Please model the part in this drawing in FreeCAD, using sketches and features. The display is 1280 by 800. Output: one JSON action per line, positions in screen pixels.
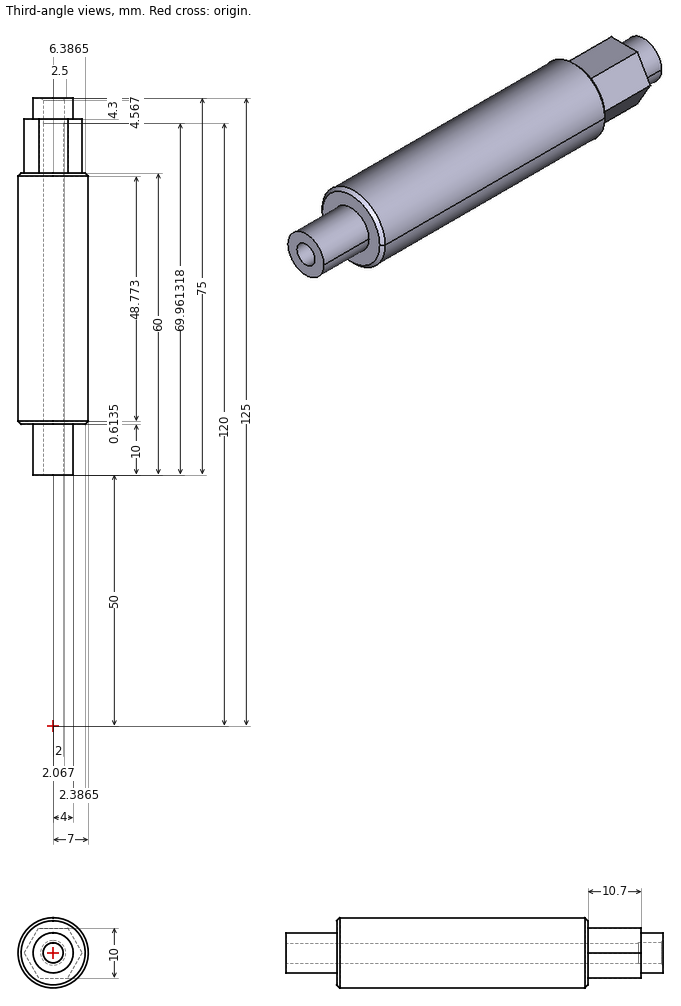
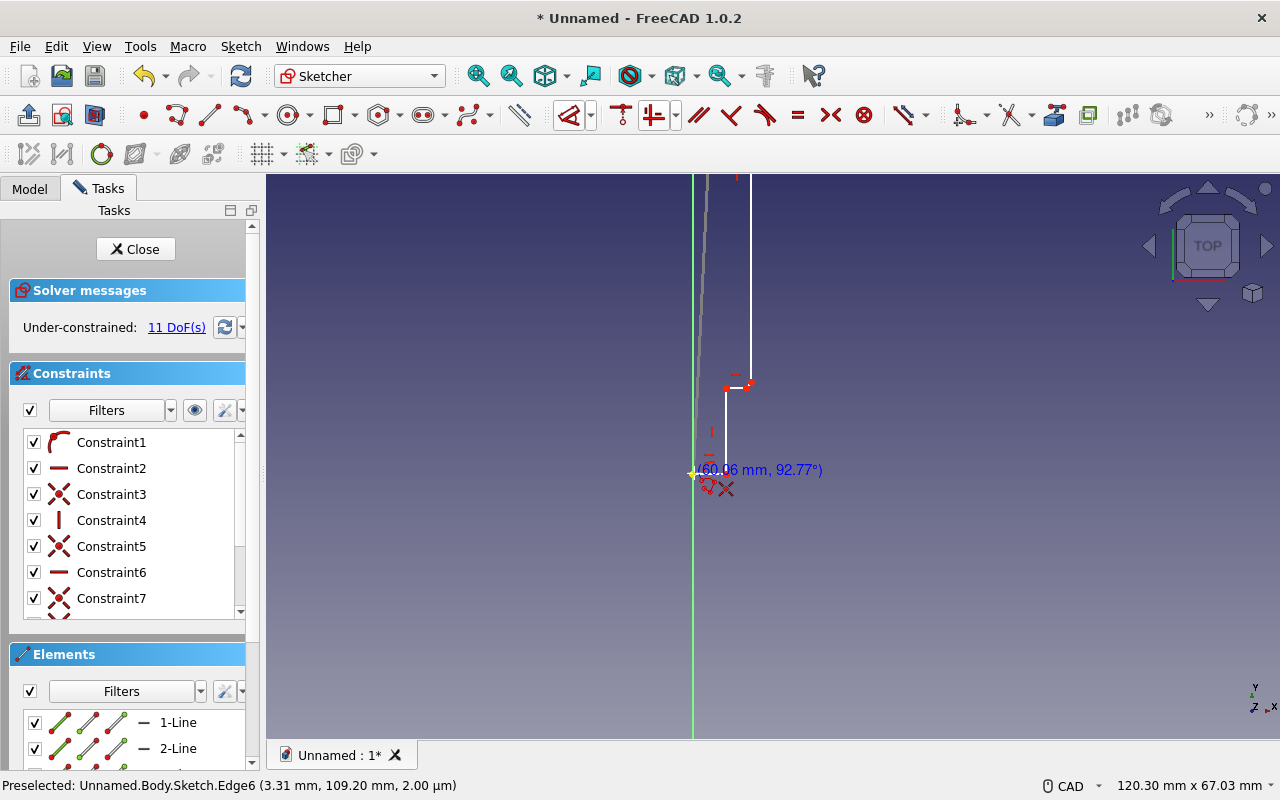
{"action": "left_click", "coordinate": [693, 474]}
{"action": "key", "text": "Escape"}
{"action": "key", "text": "Escape"}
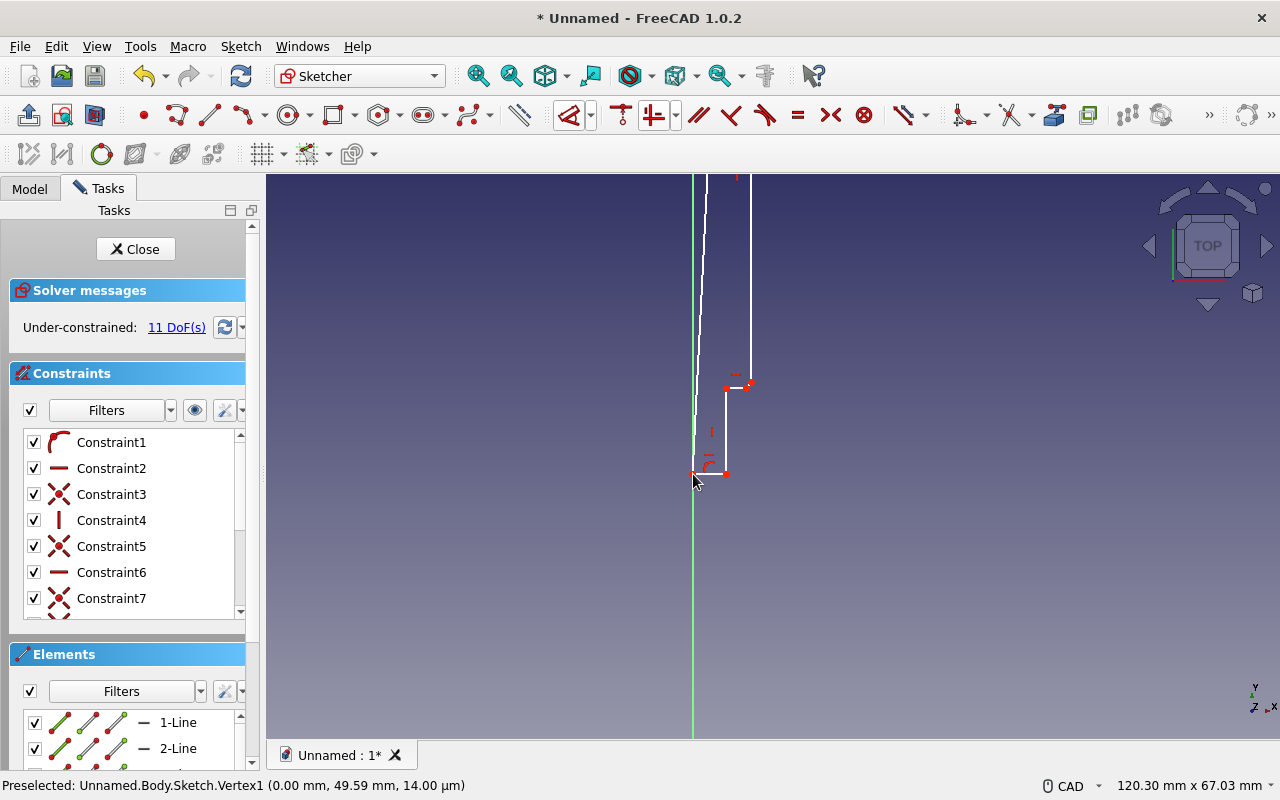
{"action": "scroll", "coordinate": [694, 473], "scroll_direction": "down", "scroll_amount": 5}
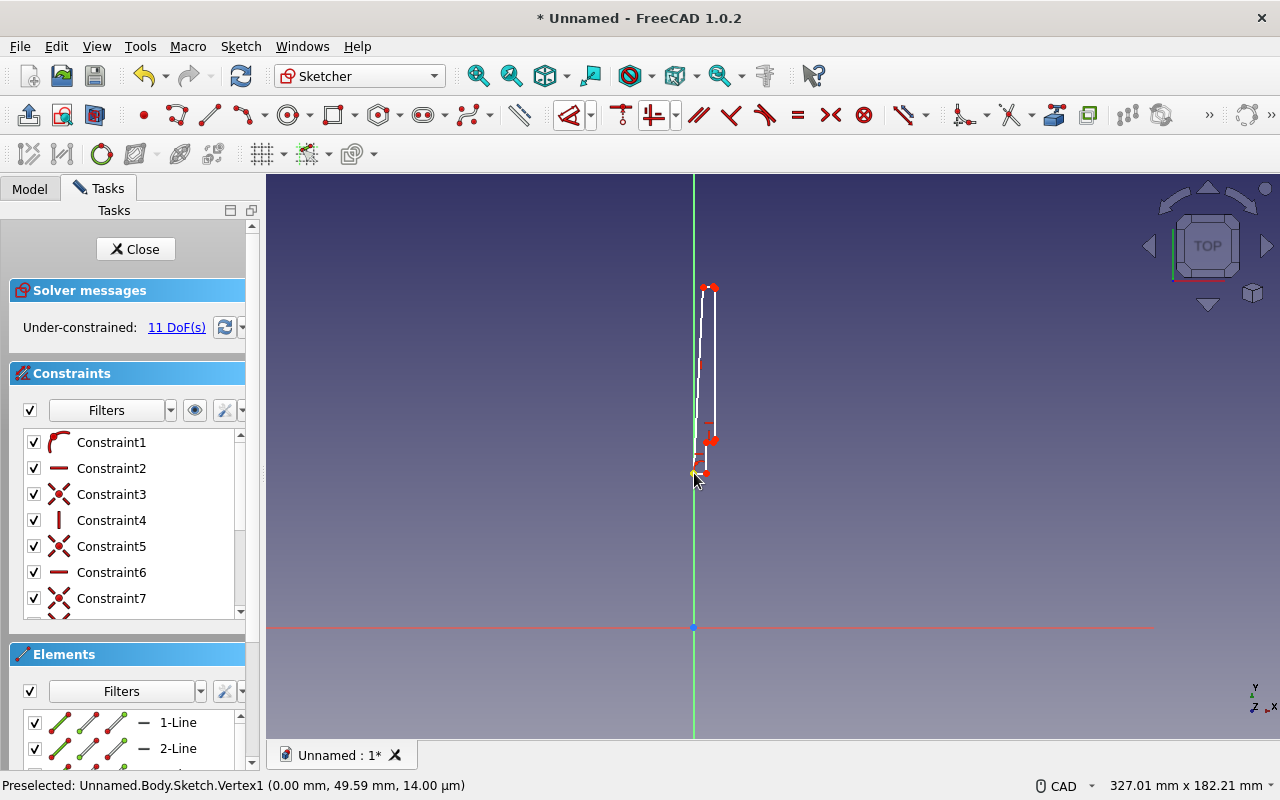
{"action": "scroll", "coordinate": [709, 287], "scroll_direction": "up", "scroll_amount": 6}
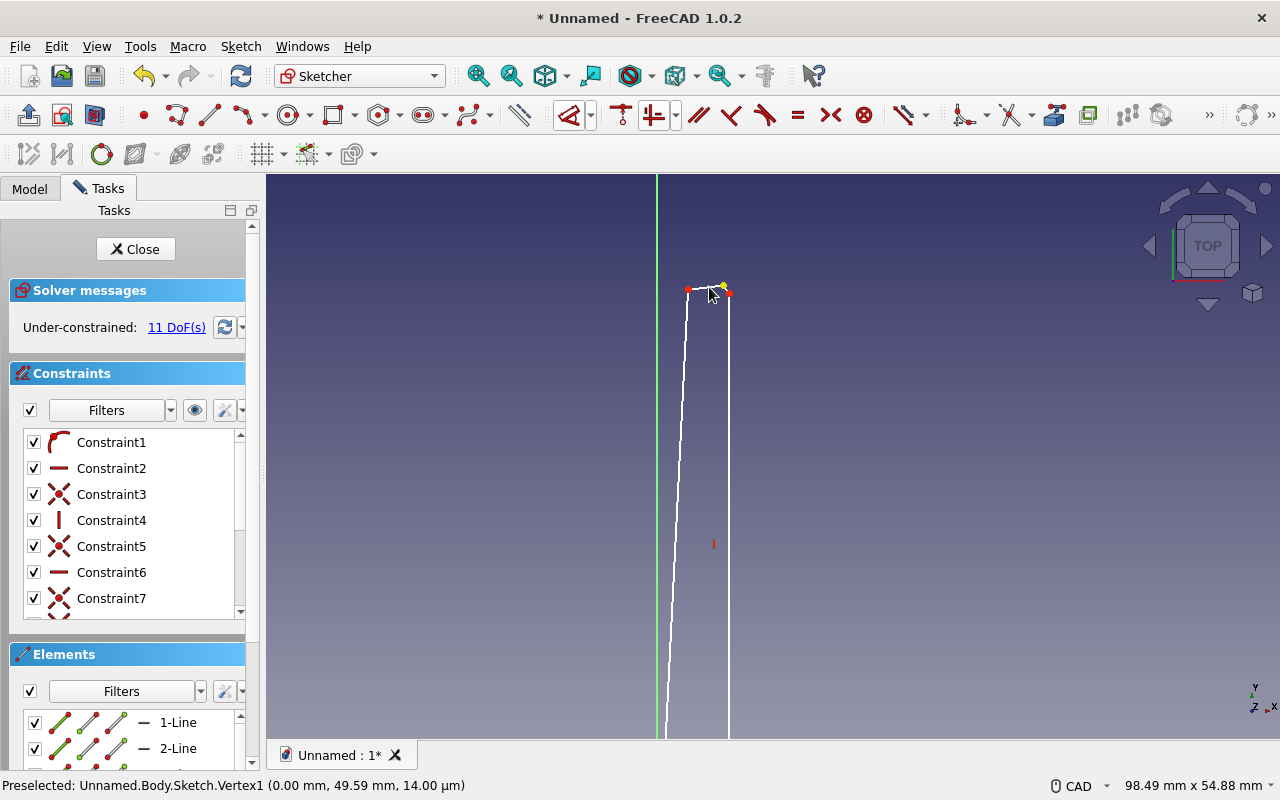
{"action": "left_click", "coordinate": [709, 287]}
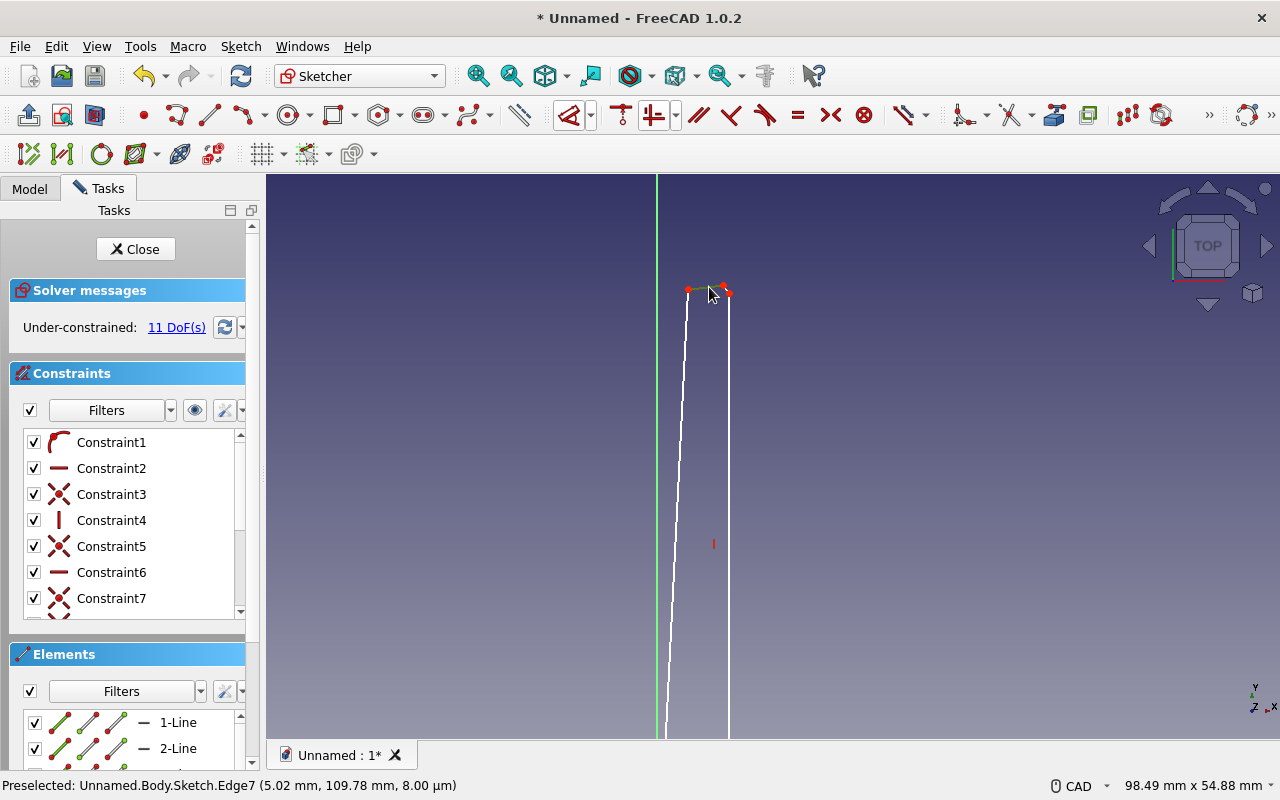
{"action": "left_click", "coordinate": [676, 116]}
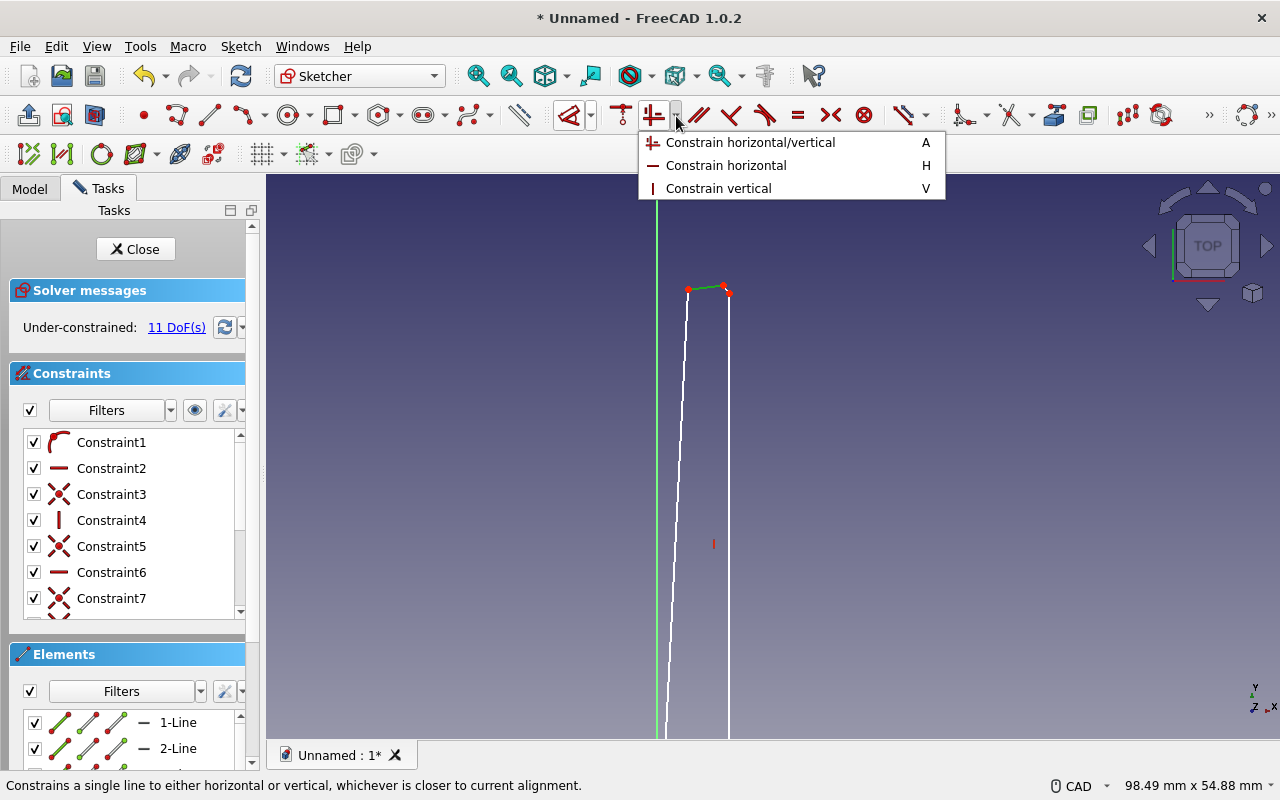
{"action": "left_click", "coordinate": [792, 166]}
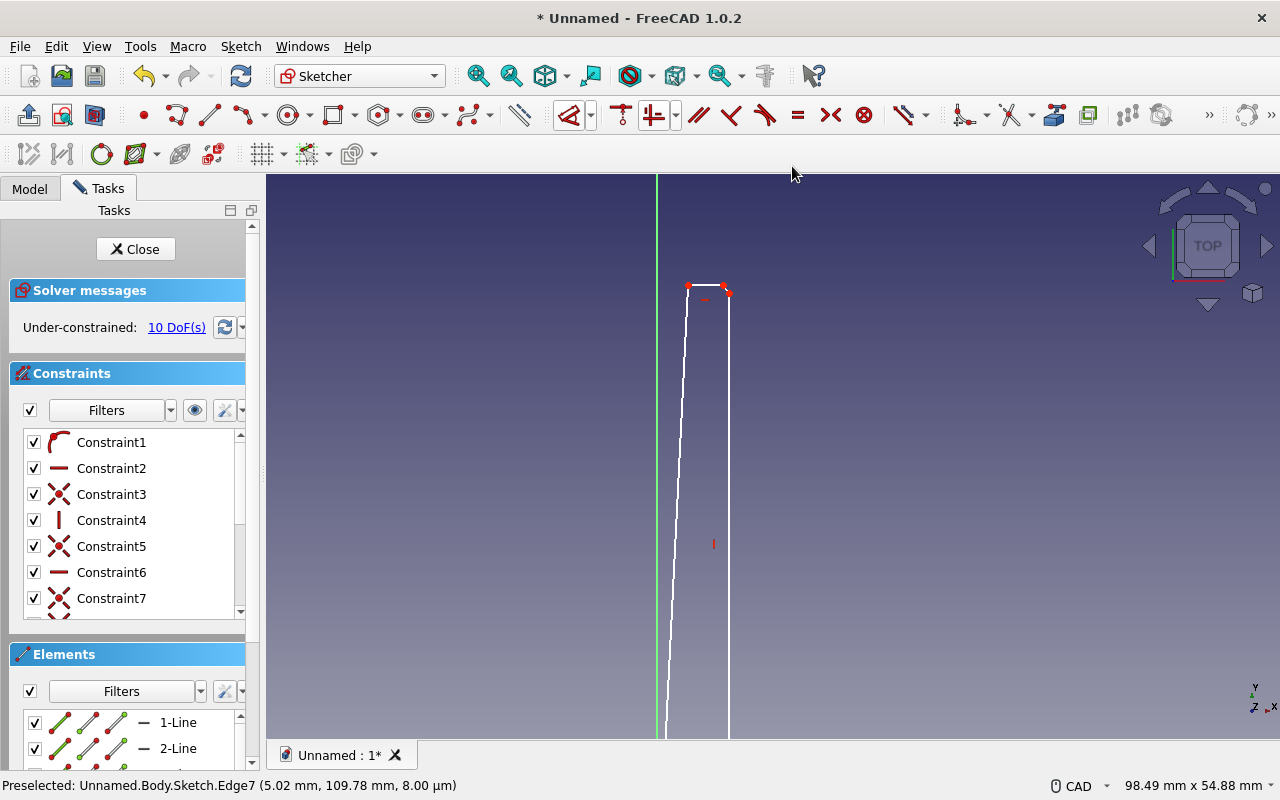
{"action": "left_click", "coordinate": [679, 472]}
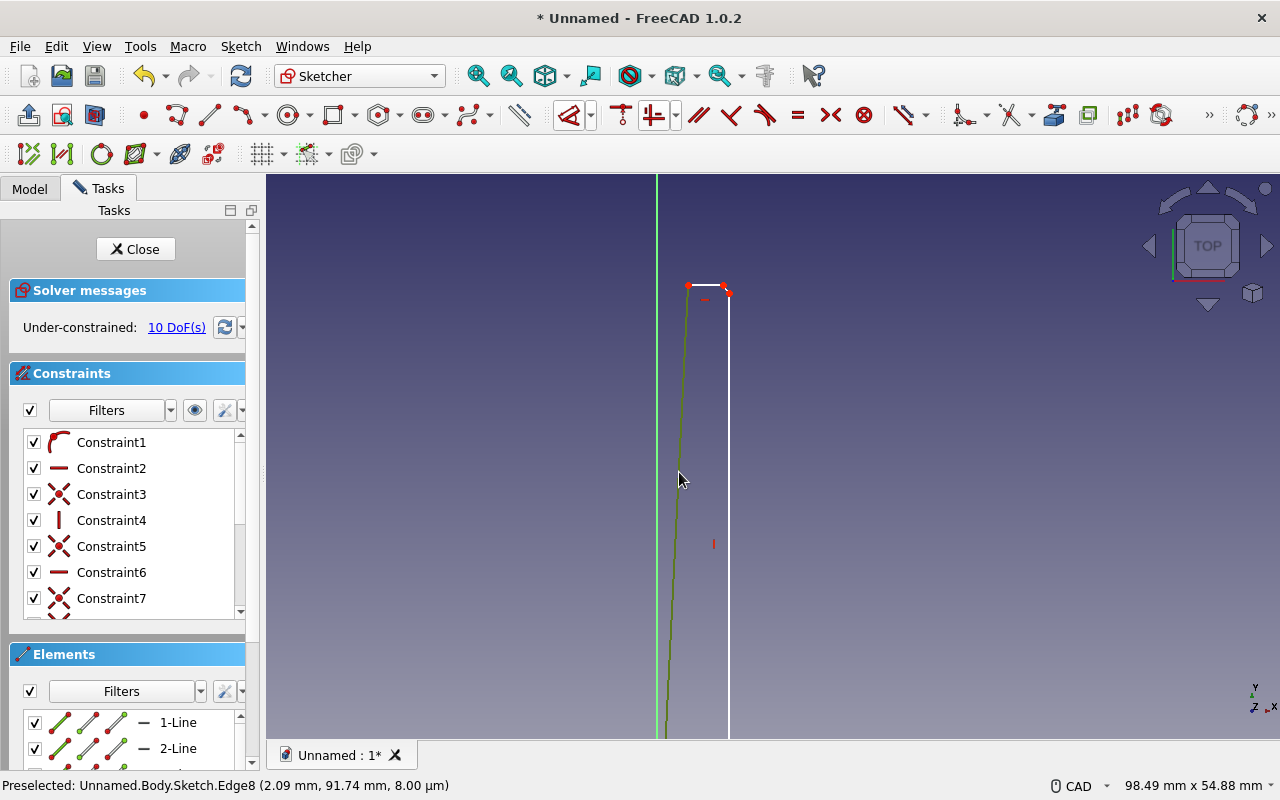
{"action": "key", "text": "v"}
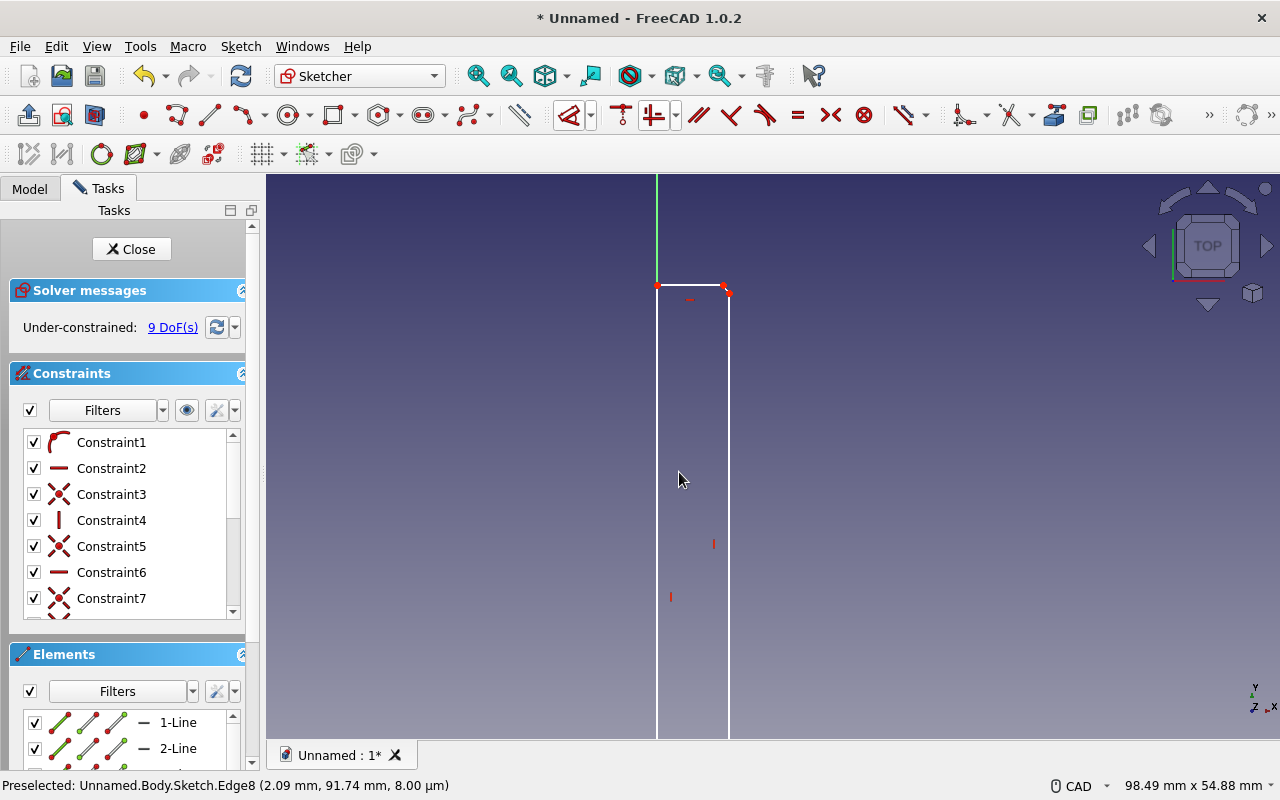
{"action": "scroll", "coordinate": [709, 286], "scroll_direction": "down", "scroll_amount": 6}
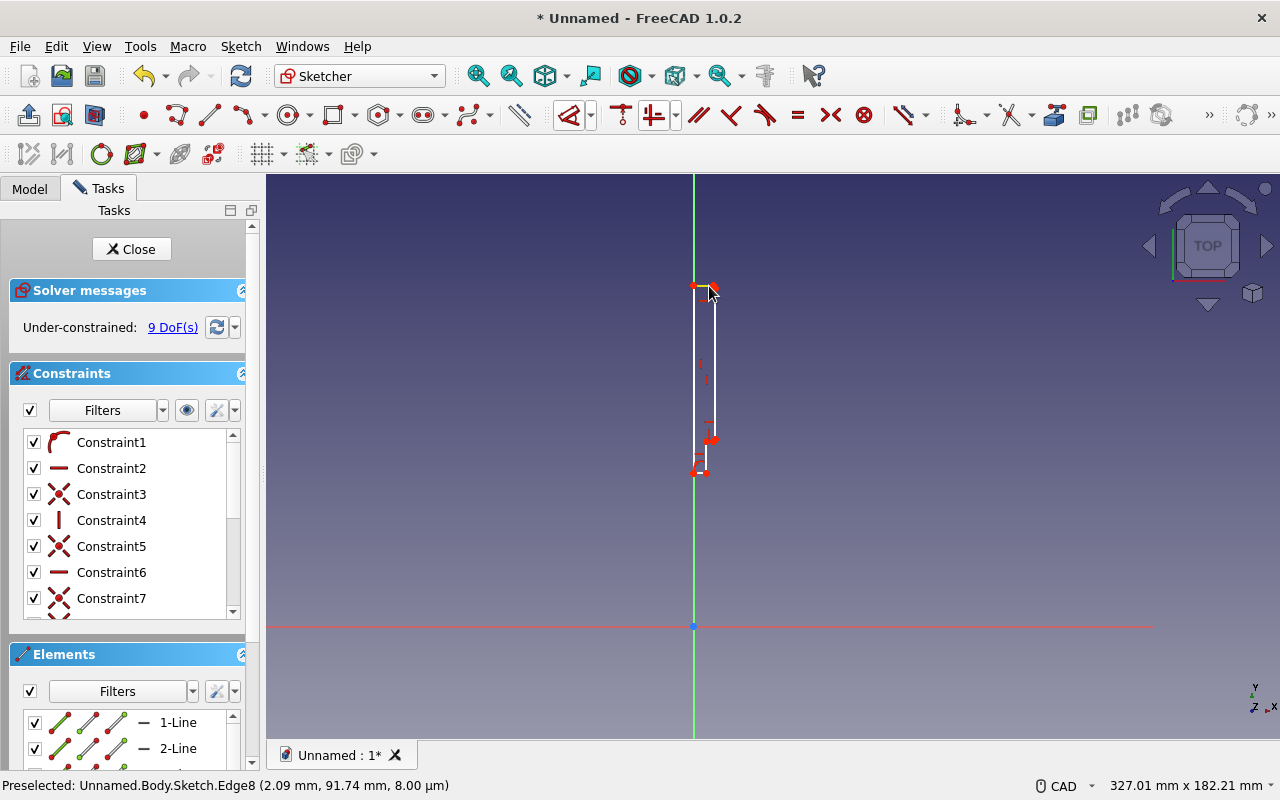
{"action": "scroll", "coordinate": [697, 473], "scroll_direction": "up", "scroll_amount": 7}